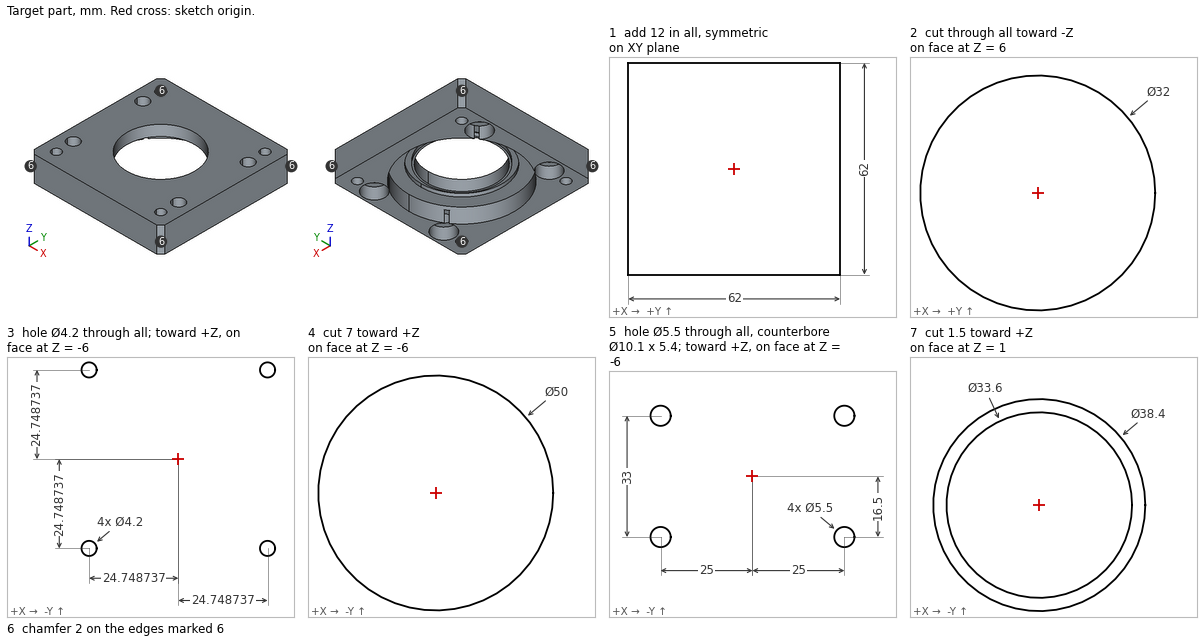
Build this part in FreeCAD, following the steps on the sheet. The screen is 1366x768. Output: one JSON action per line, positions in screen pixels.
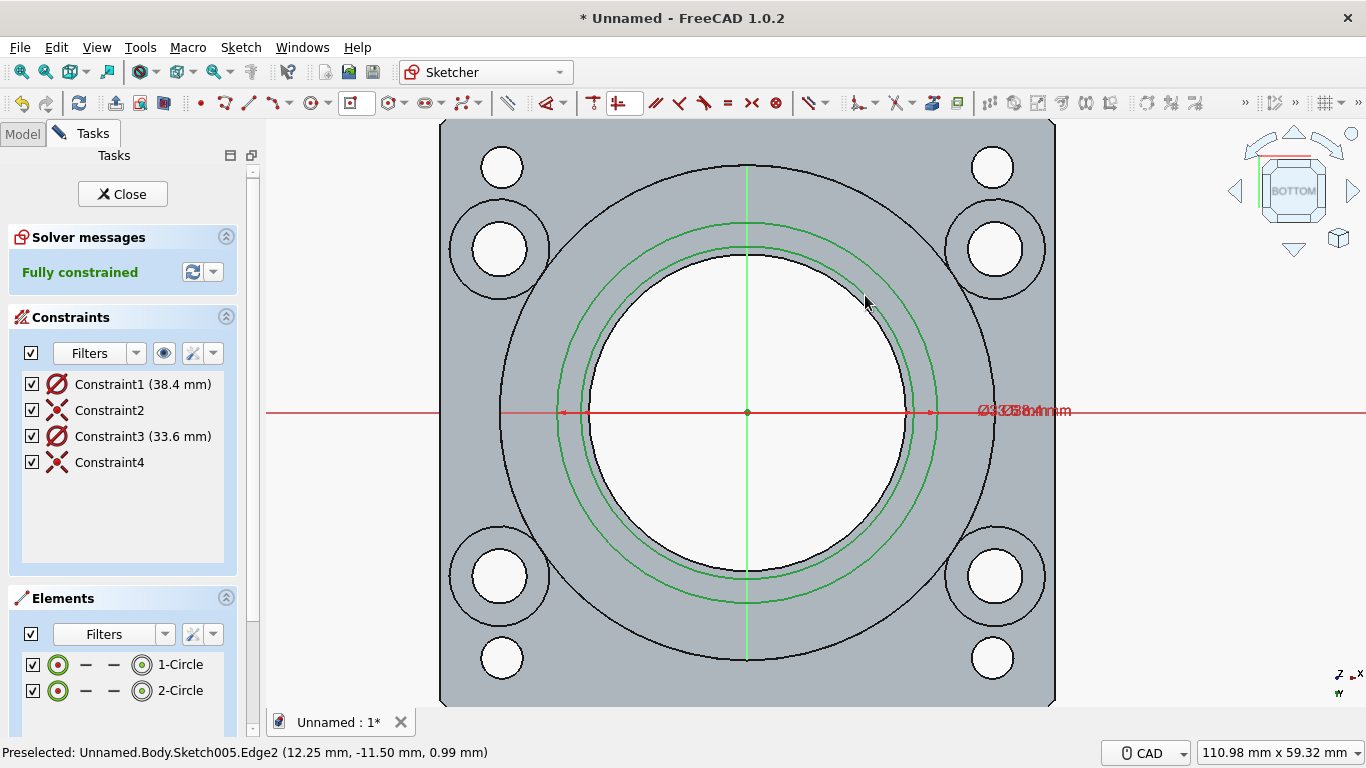
{"action": "left_click", "coordinate": [123, 194]}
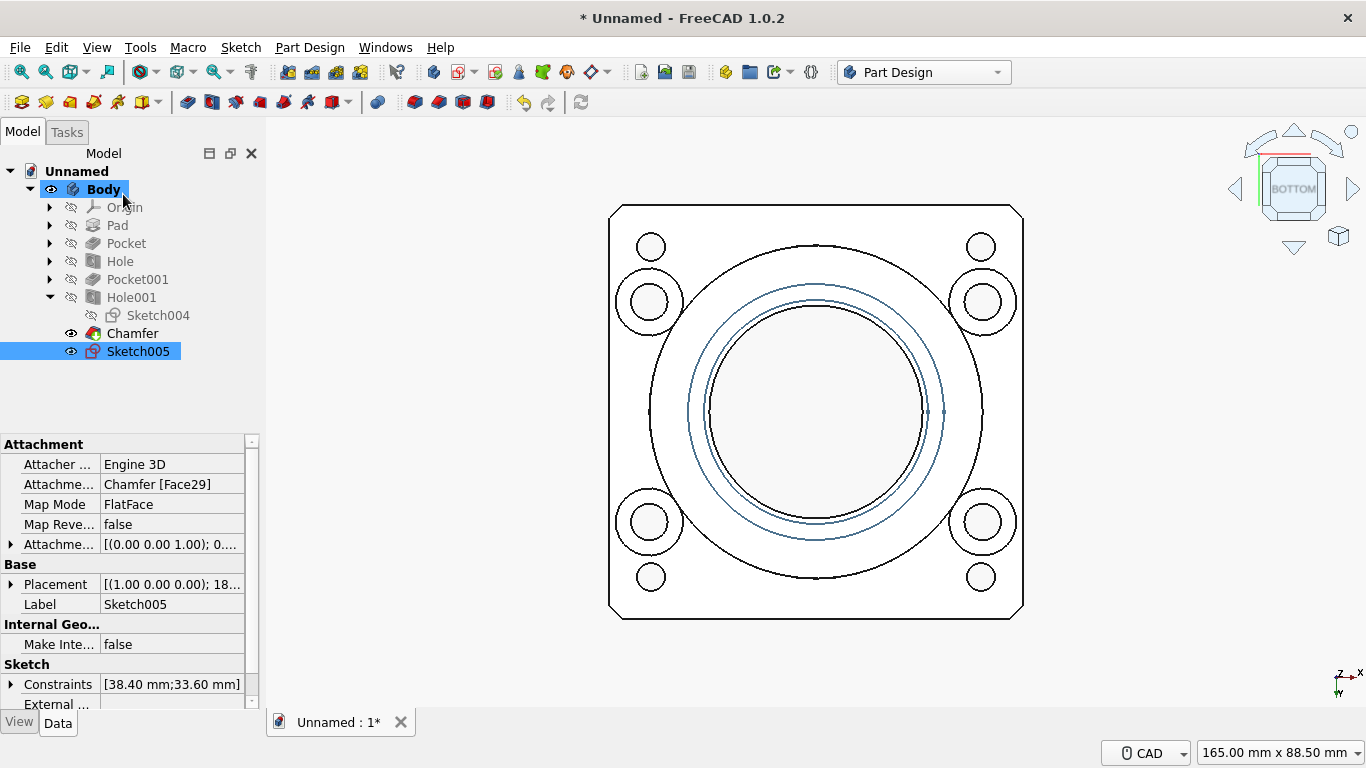
{"action": "left_click", "coordinate": [188, 102]}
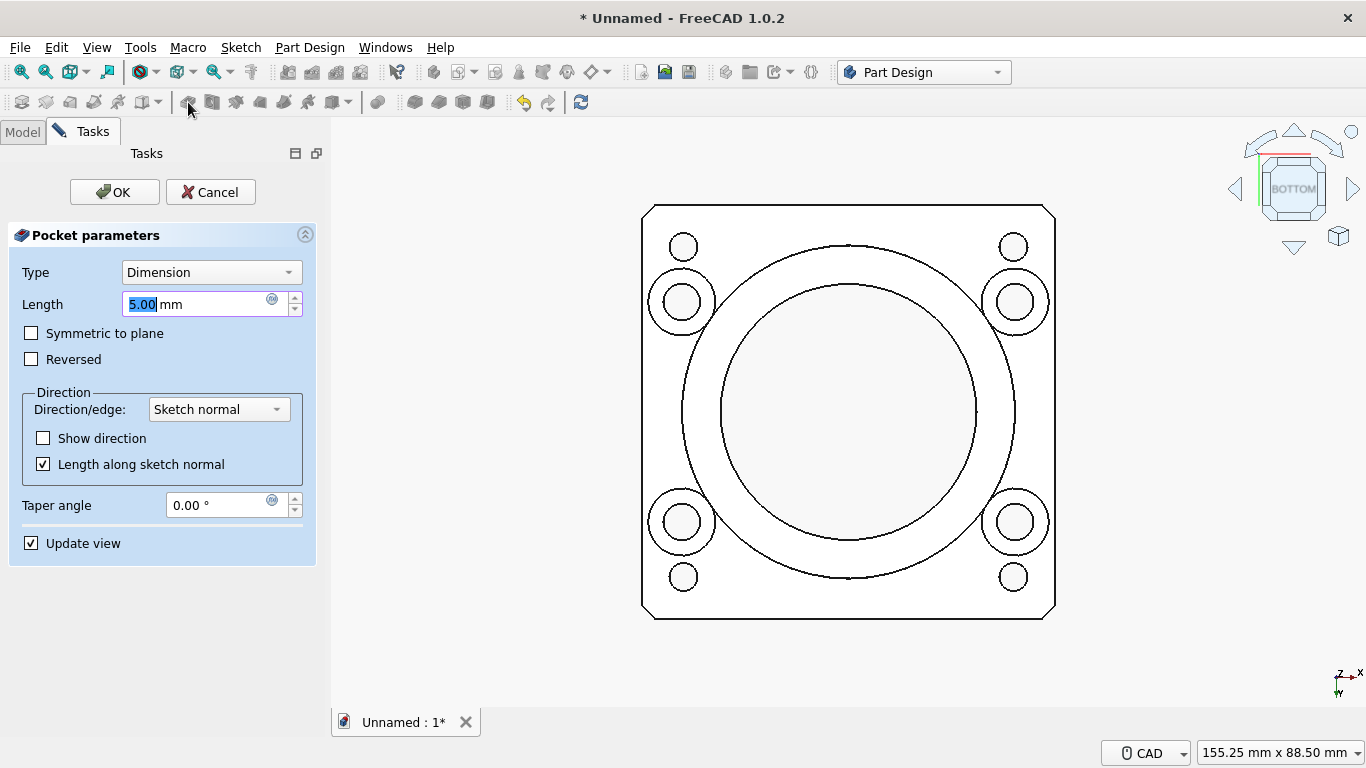
{"action": "type", "text": "1.5"}
{"action": "key", "text": "Tab"}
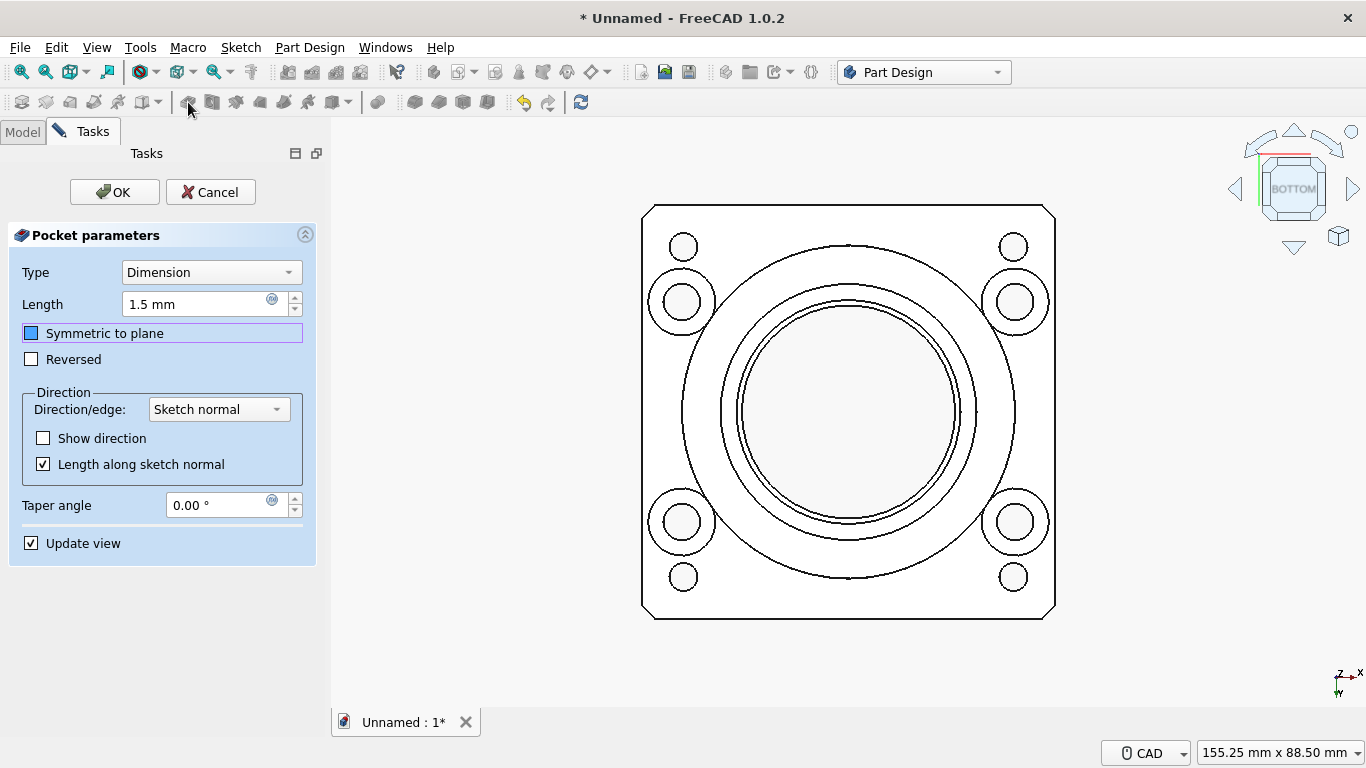
{"action": "left_click", "coordinate": [115, 192]}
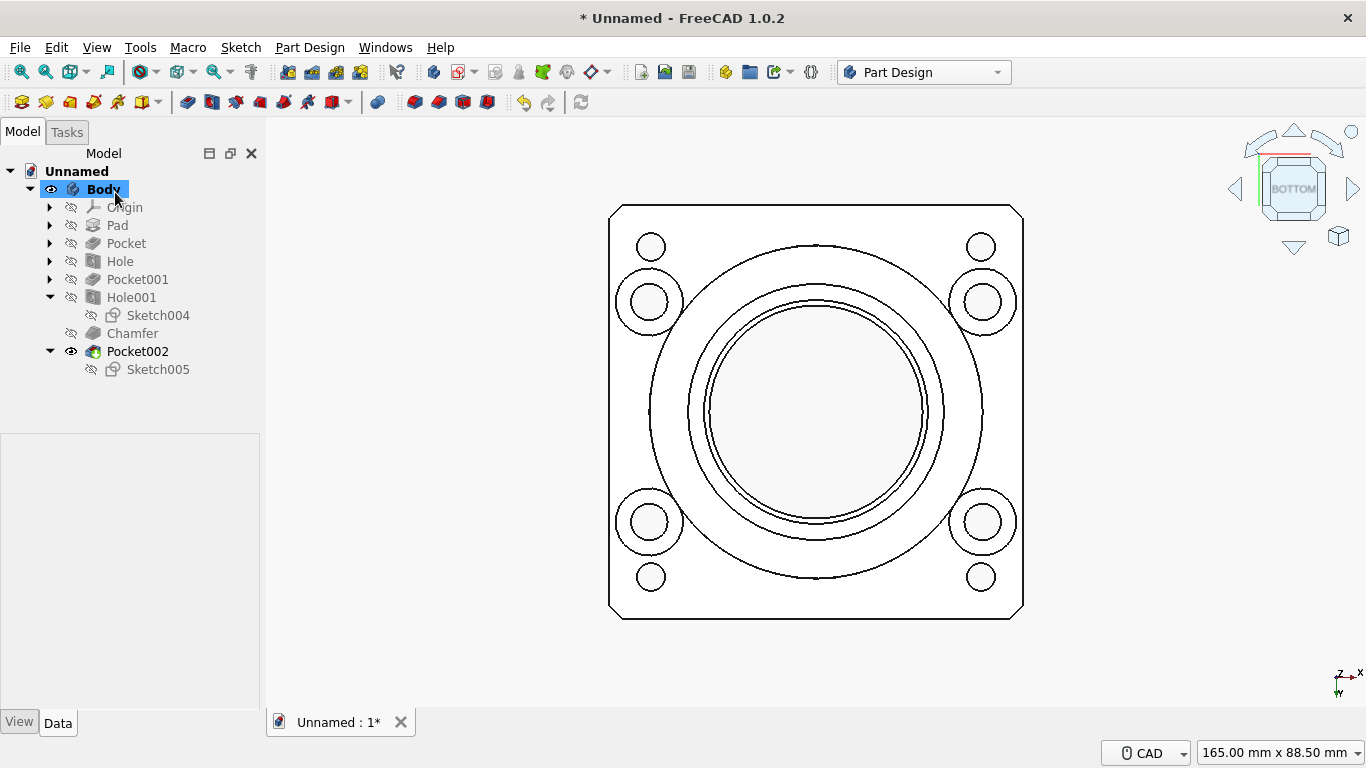
{"action": "key", "text": "0"}